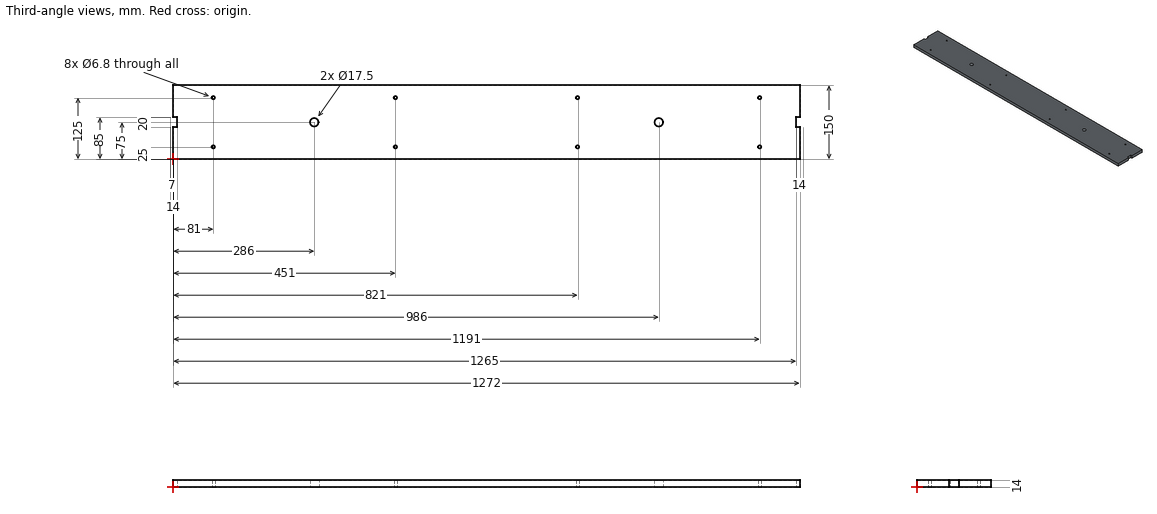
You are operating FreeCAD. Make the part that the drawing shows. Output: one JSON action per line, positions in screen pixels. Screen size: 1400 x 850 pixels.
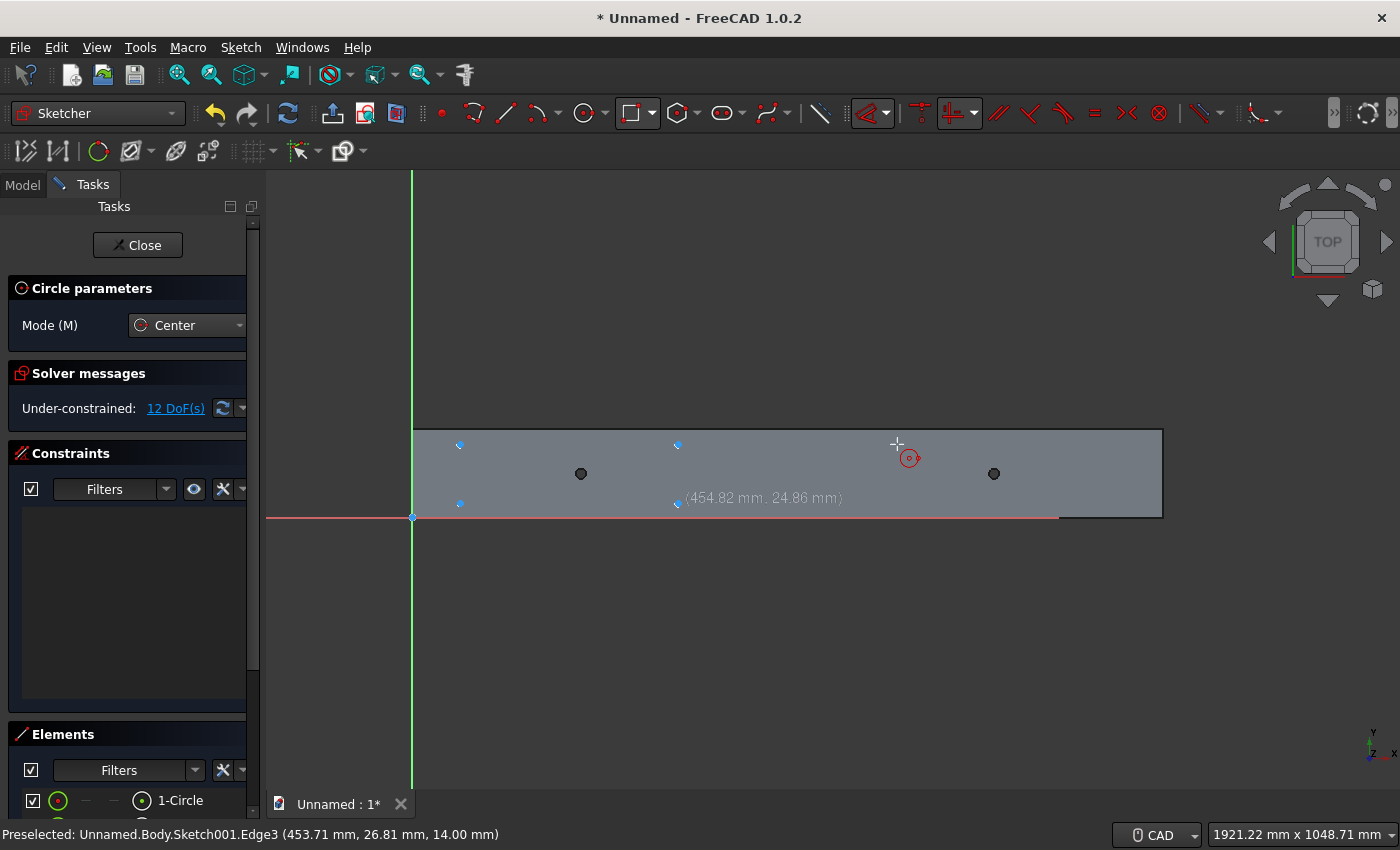
{"action": "left_click", "coordinate": [897, 444]}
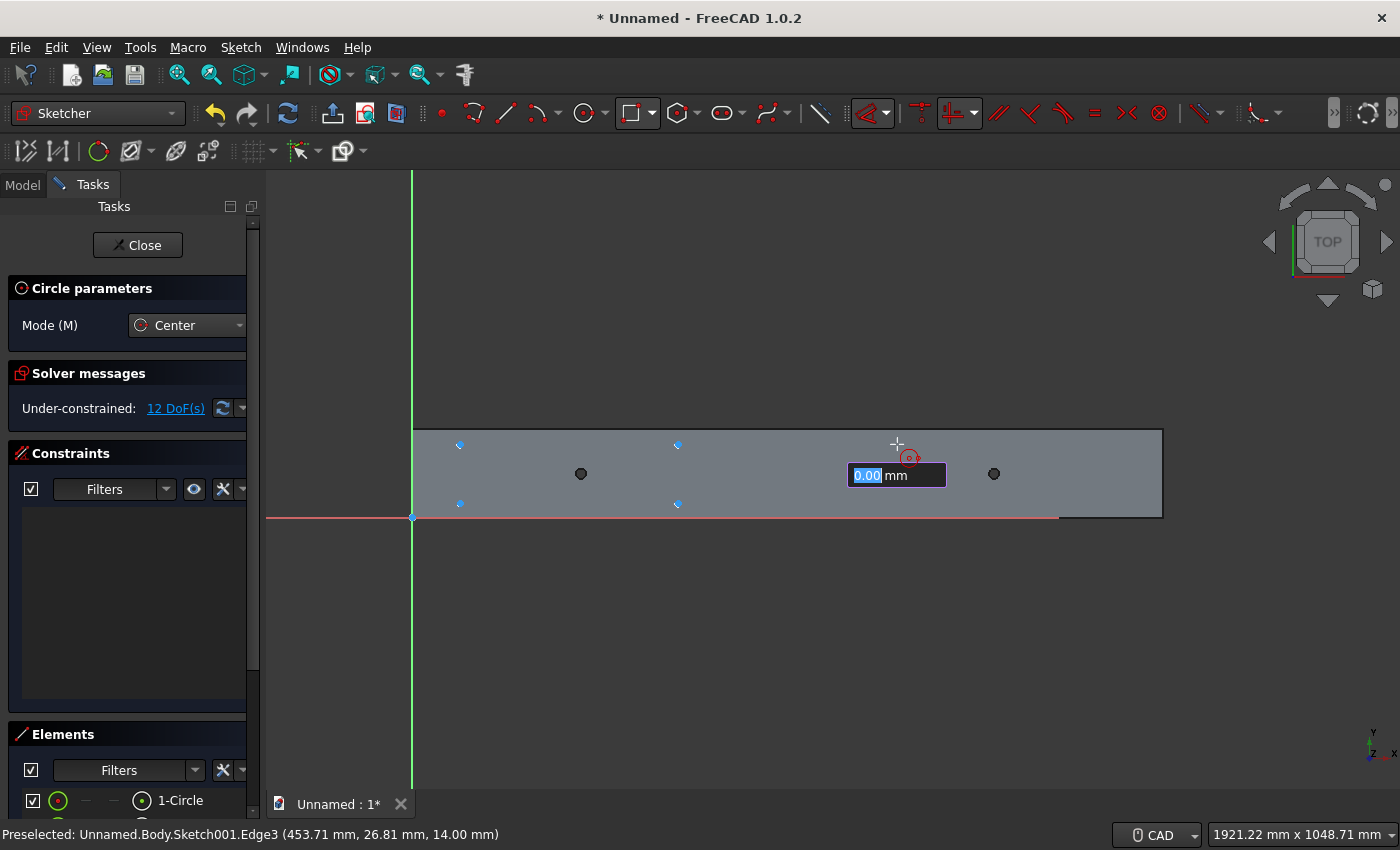
{"action": "scroll", "coordinate": [898, 443], "scroll_direction": "up", "scroll_amount": 11}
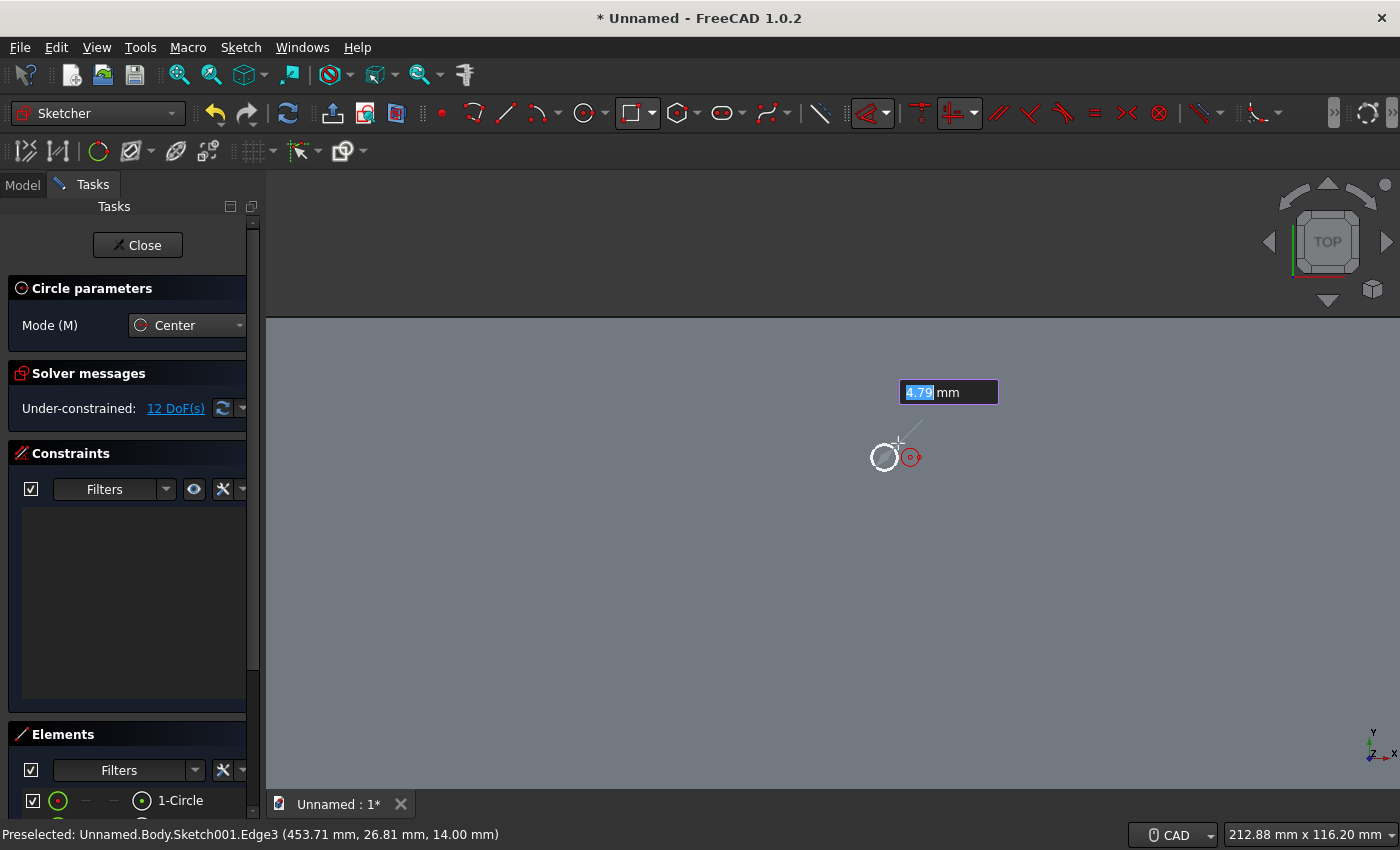
{"action": "left_click", "coordinate": [895, 437]}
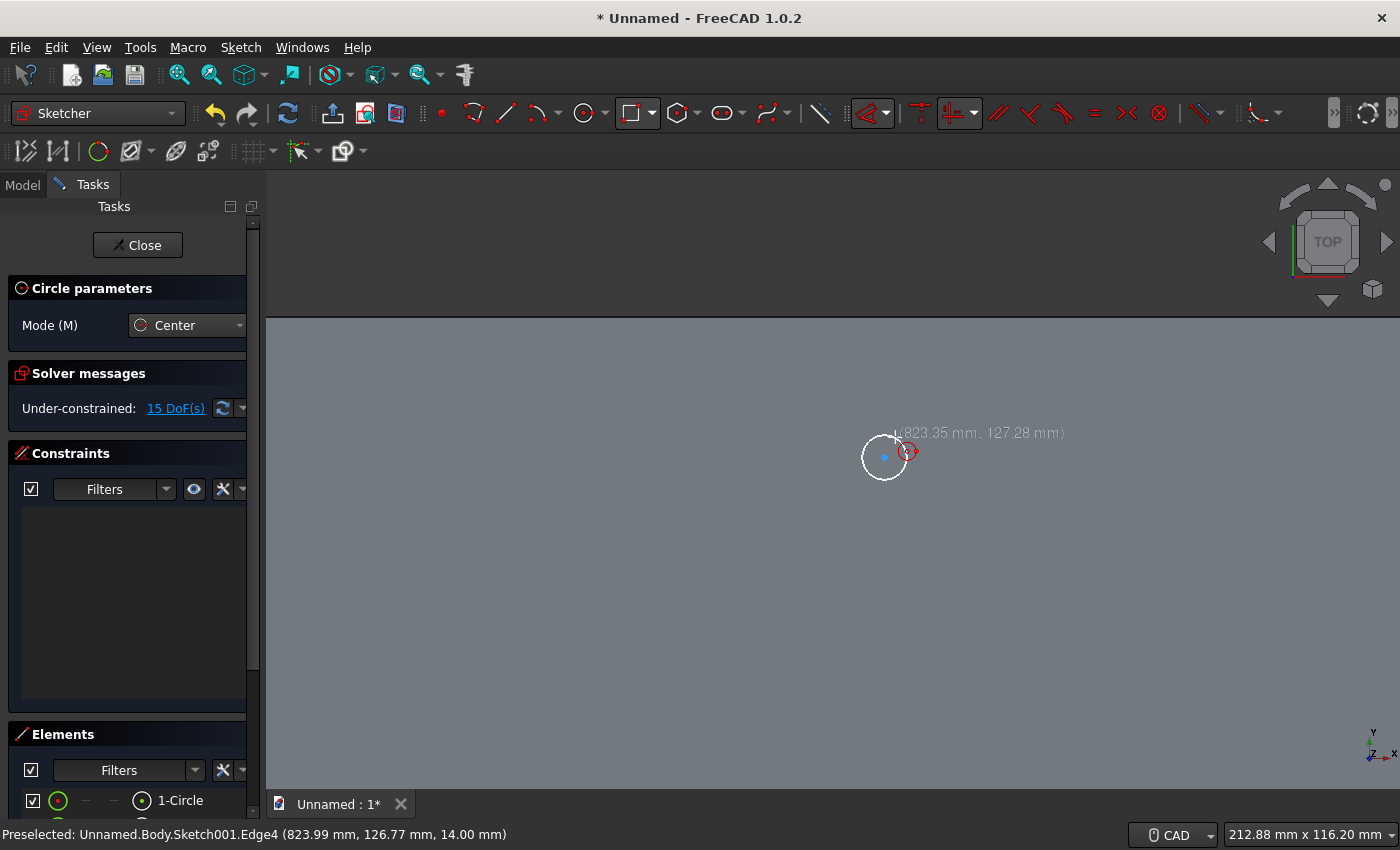
{"action": "scroll", "coordinate": [898, 443], "scroll_direction": "down", "scroll_amount": 11}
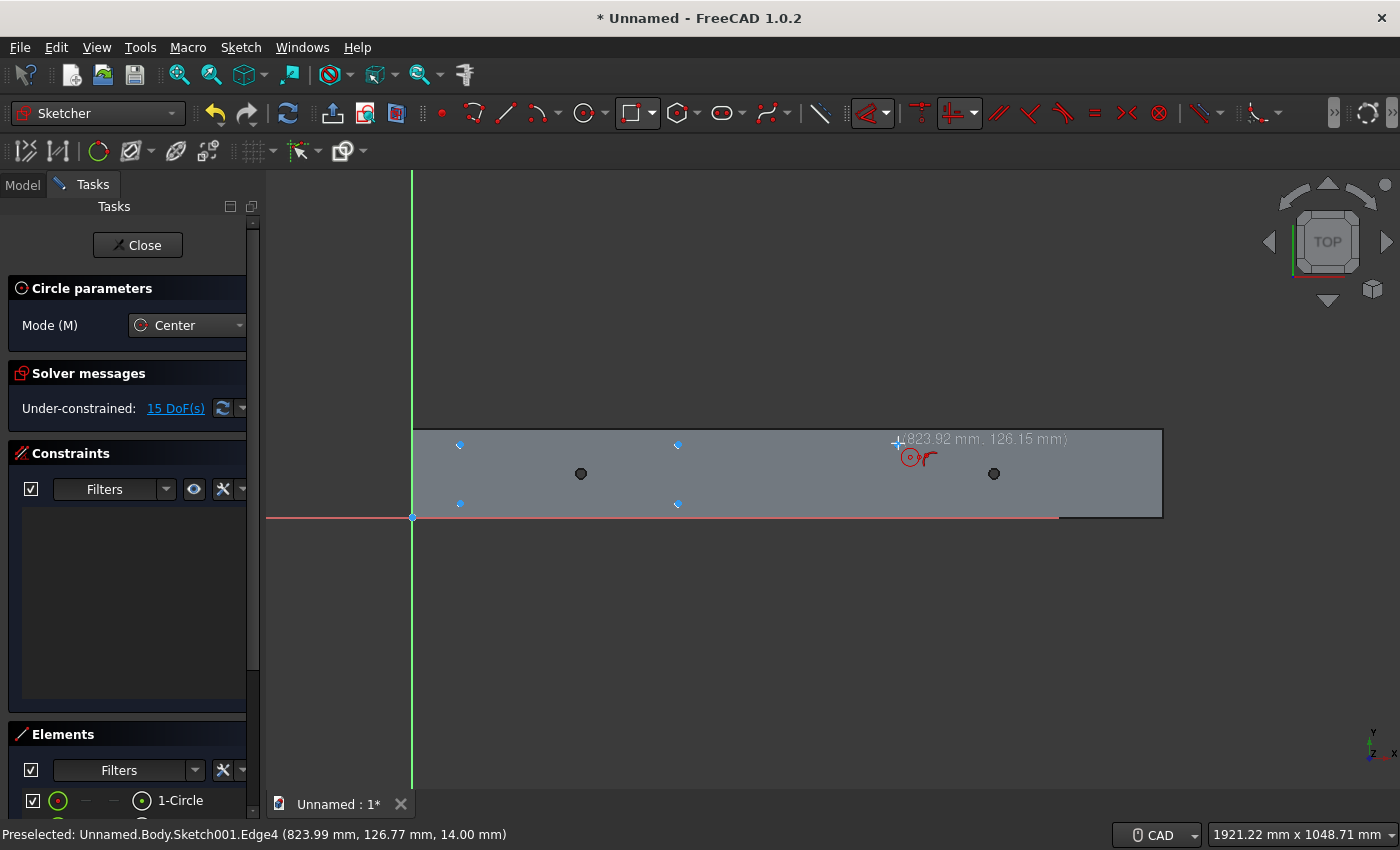
{"action": "scroll", "coordinate": [897, 503], "scroll_direction": "up", "scroll_amount": 13}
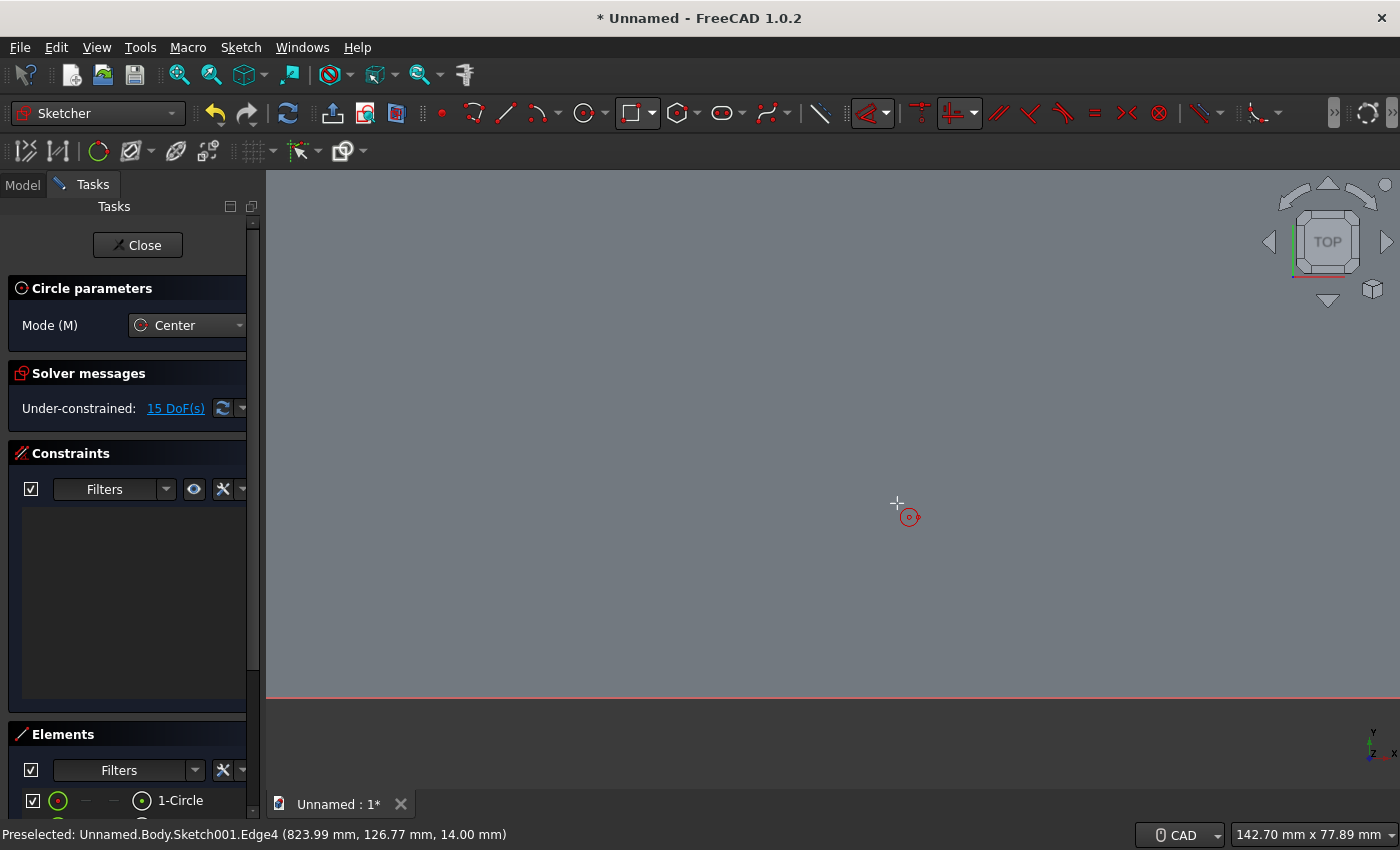
{"action": "scroll", "coordinate": [897, 503], "scroll_direction": "down", "scroll_amount": 13}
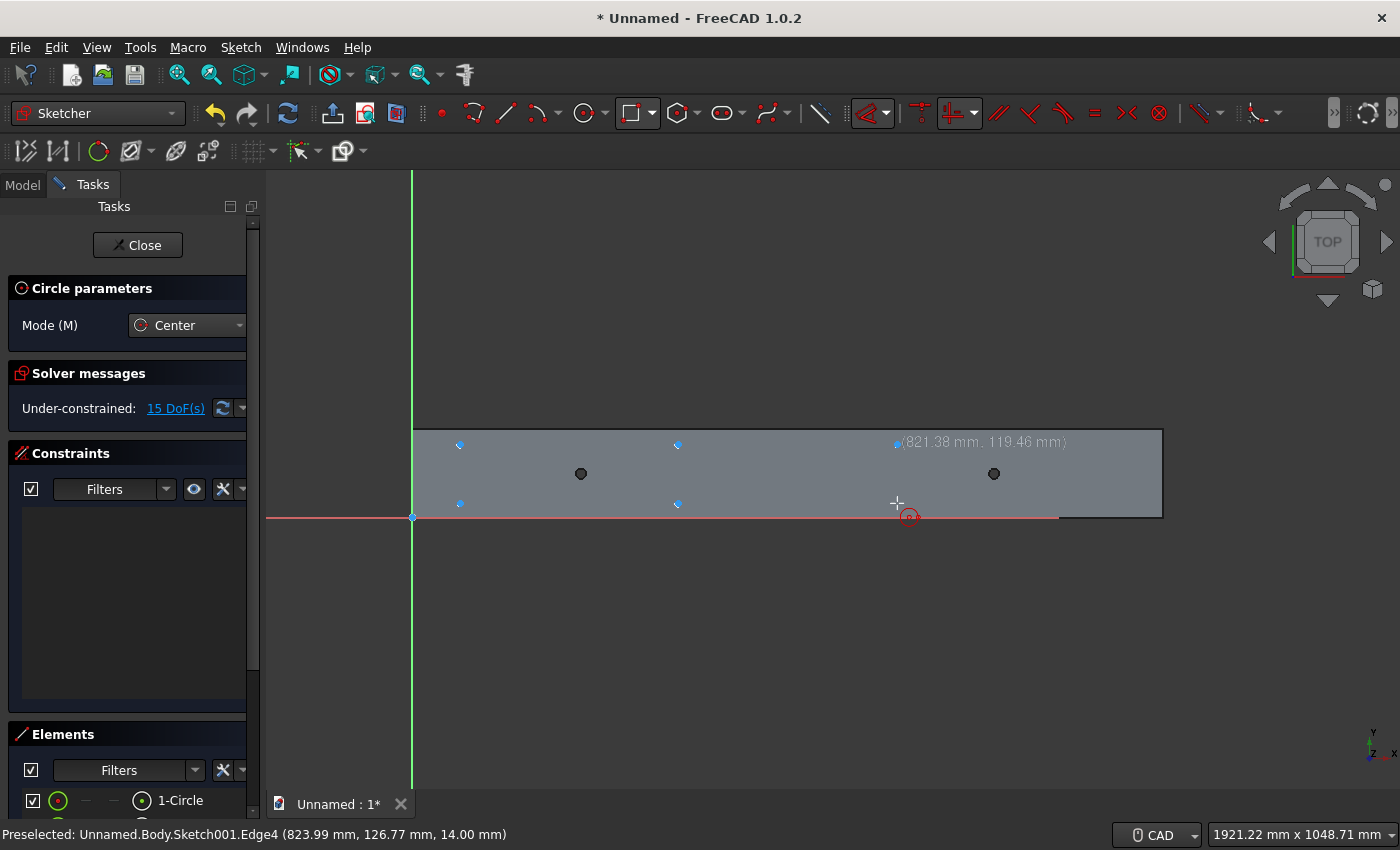
{"action": "left_click", "coordinate": [897, 503]}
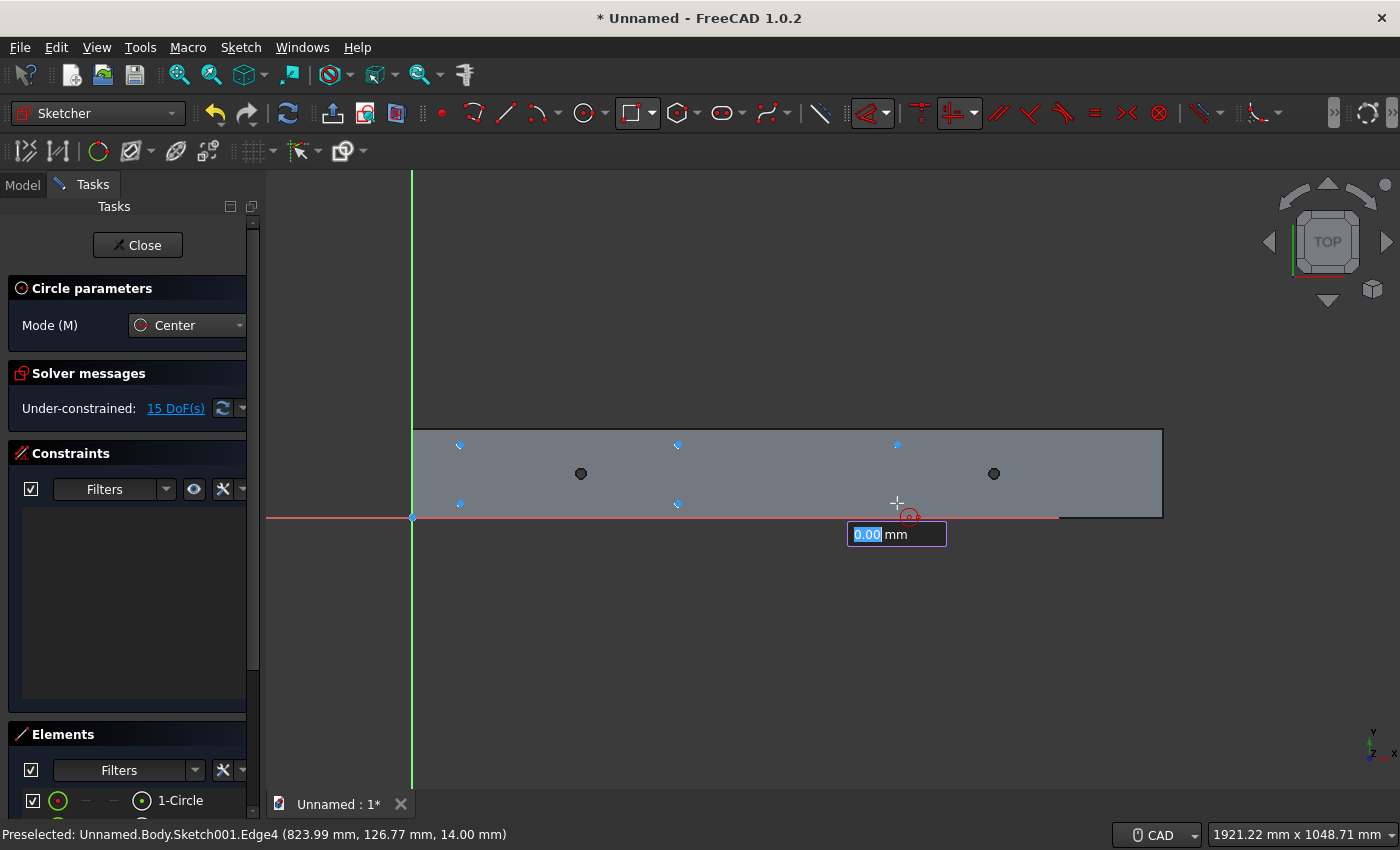
{"action": "scroll", "coordinate": [898, 502], "scroll_direction": "up", "scroll_amount": 11}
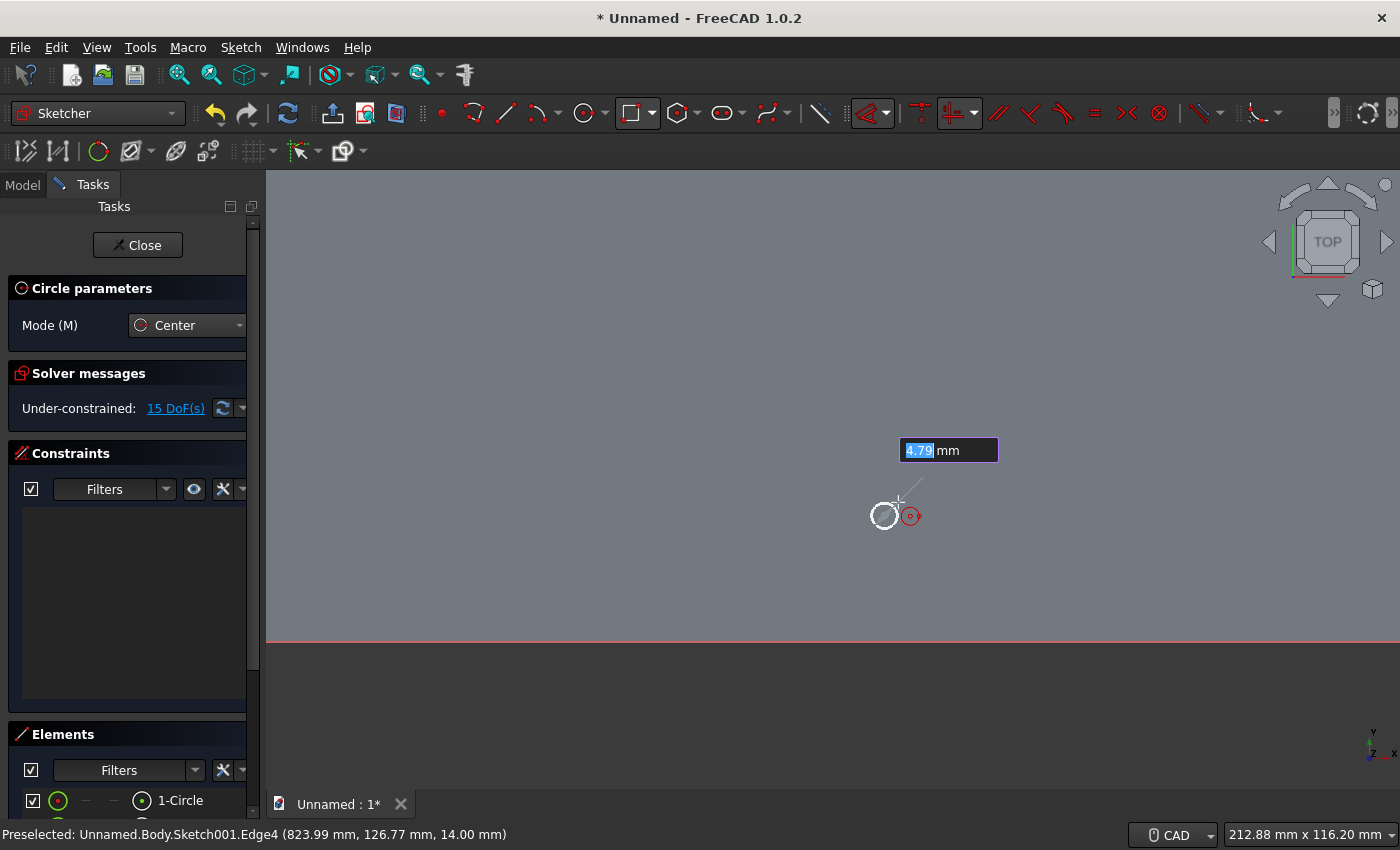
{"action": "left_click", "coordinate": [895, 496]}